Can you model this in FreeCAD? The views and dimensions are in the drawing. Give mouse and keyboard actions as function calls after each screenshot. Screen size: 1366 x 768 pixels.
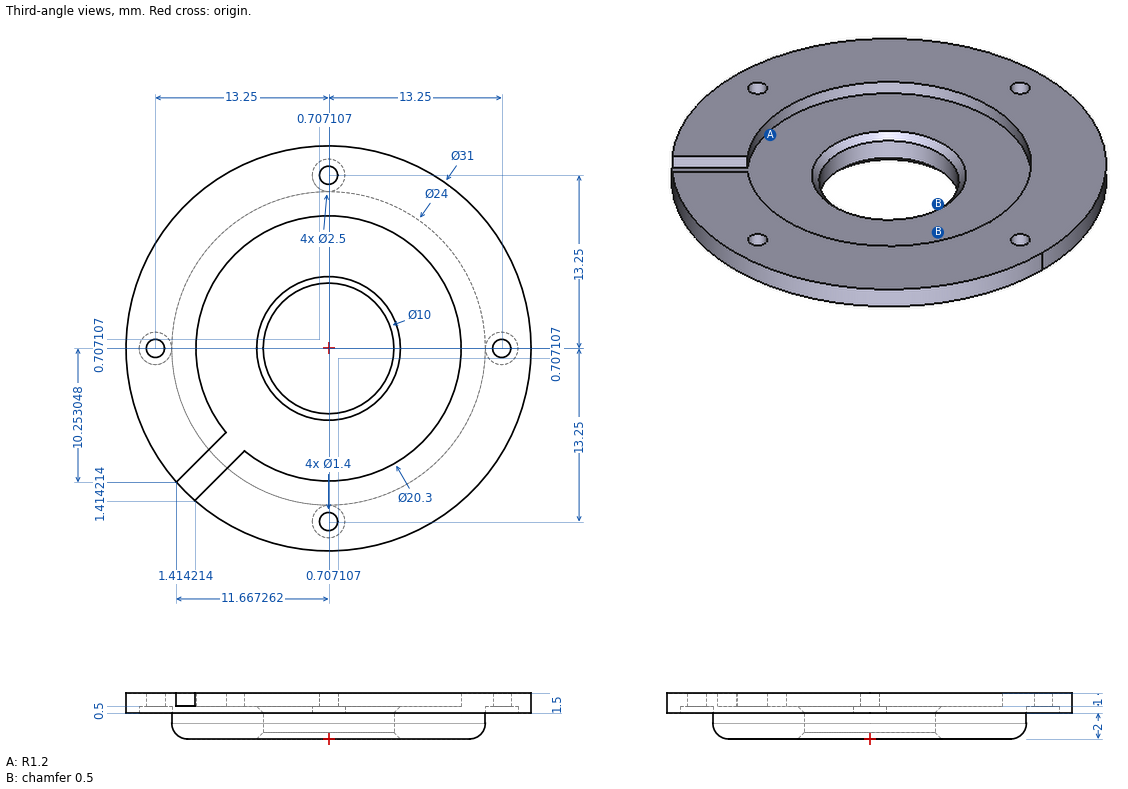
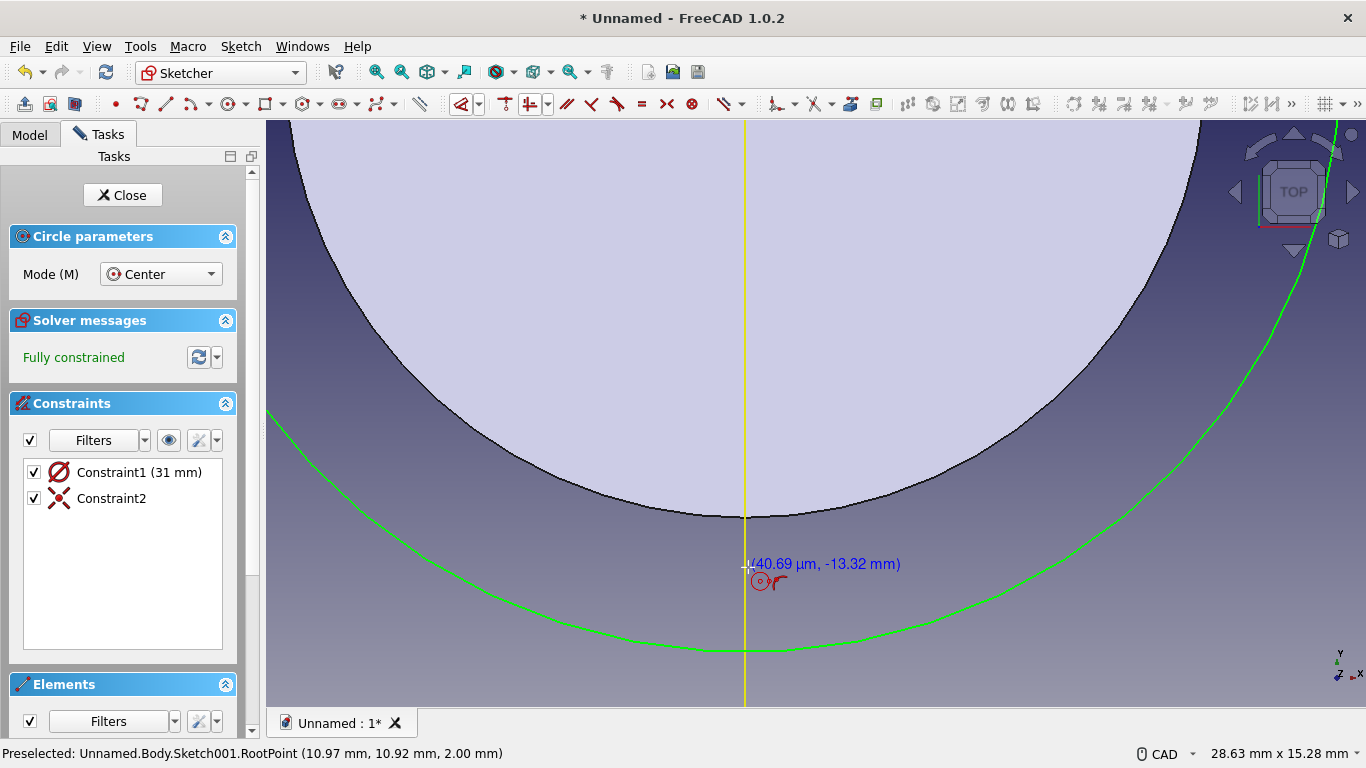
click(745, 566)
move(764, 547)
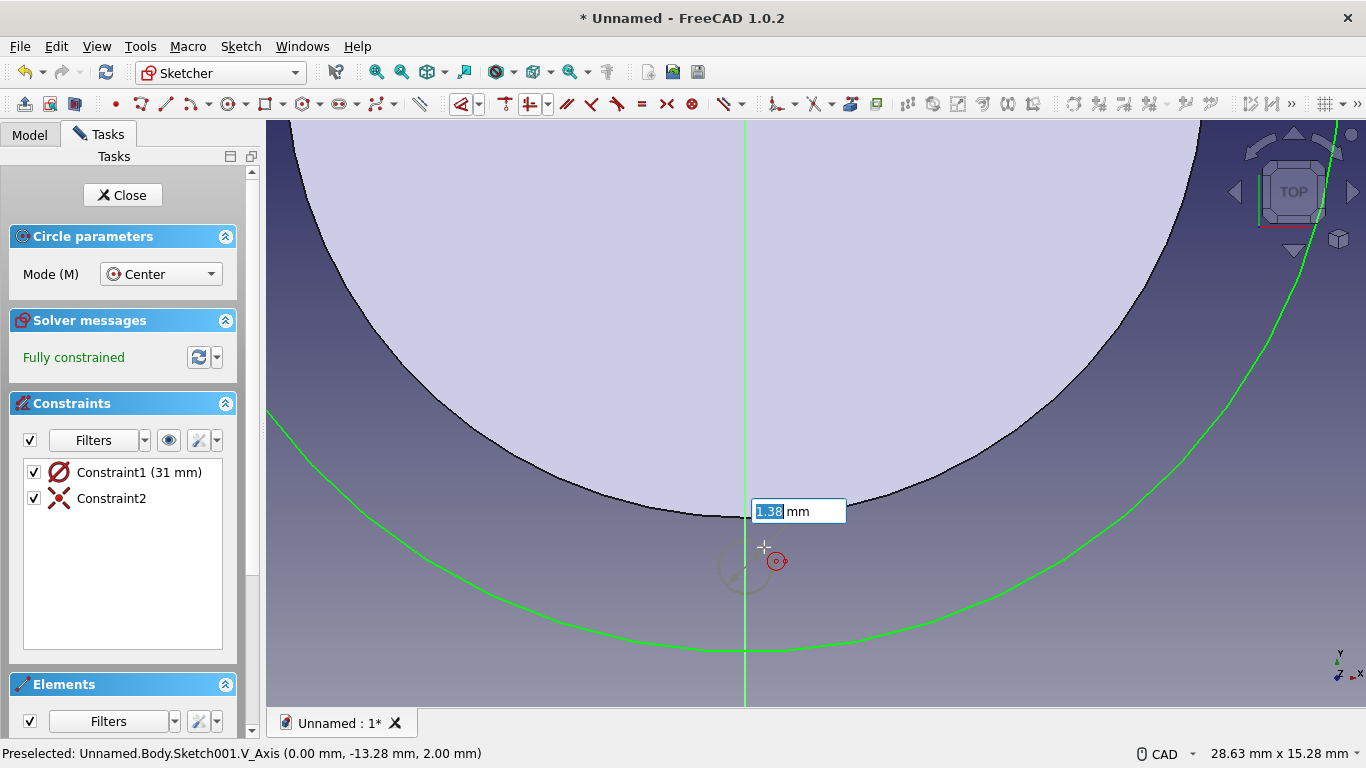
text(1.4)
key(Return)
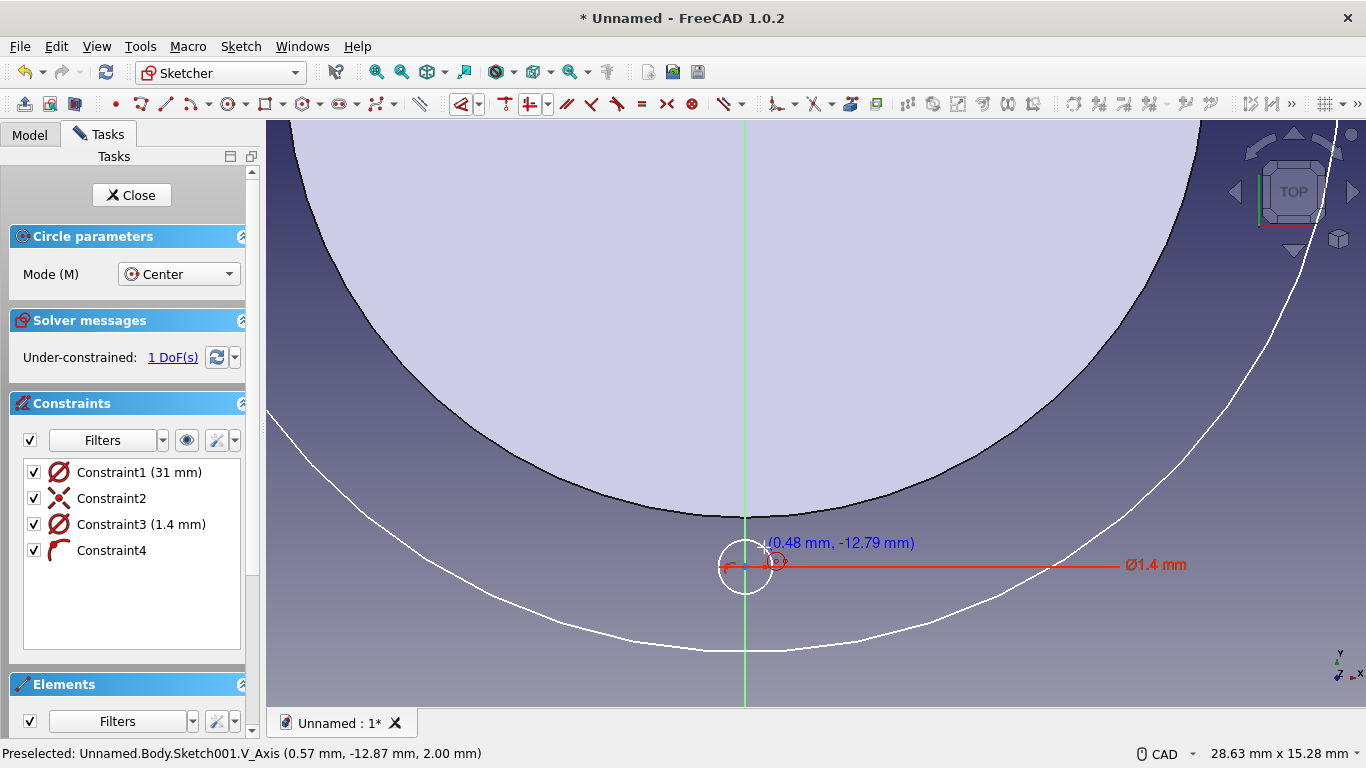
scroll(748, 567, down, 6)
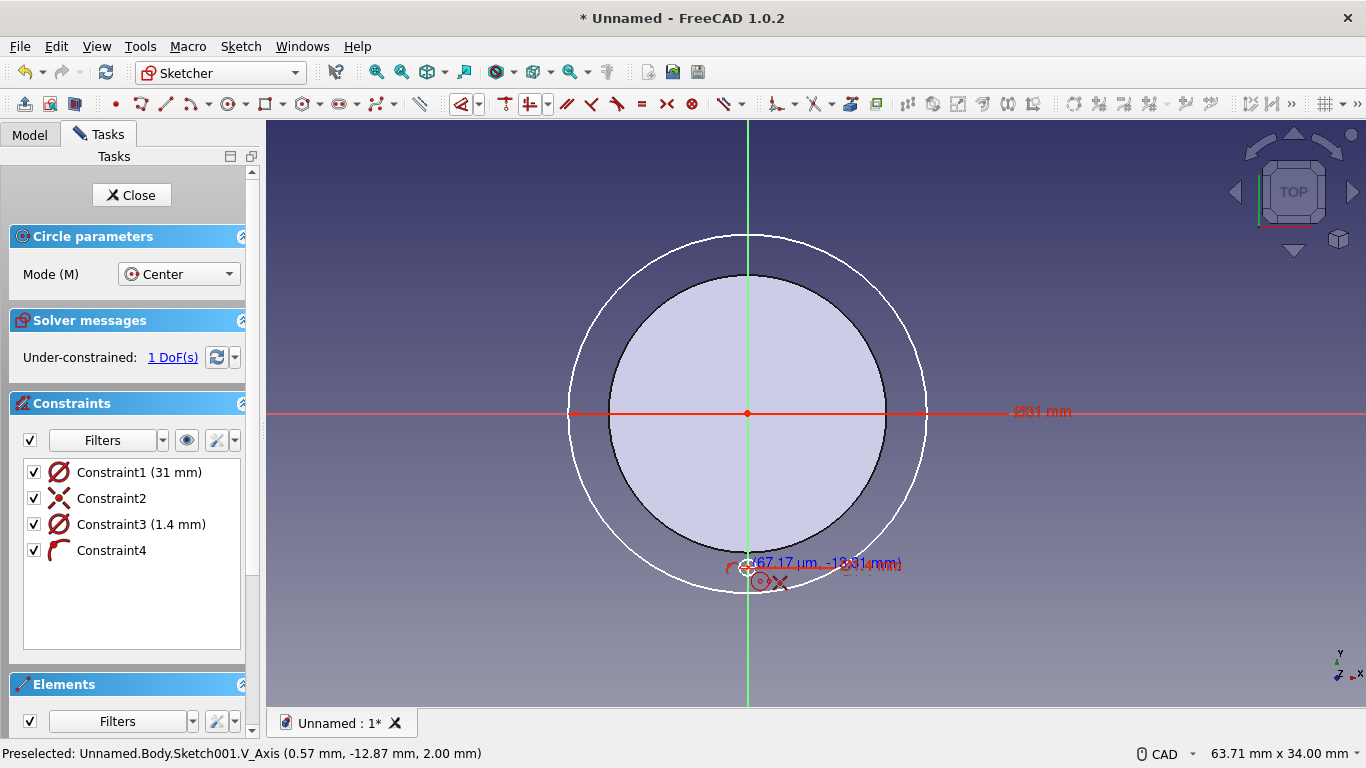
scroll(594, 414, up, 6)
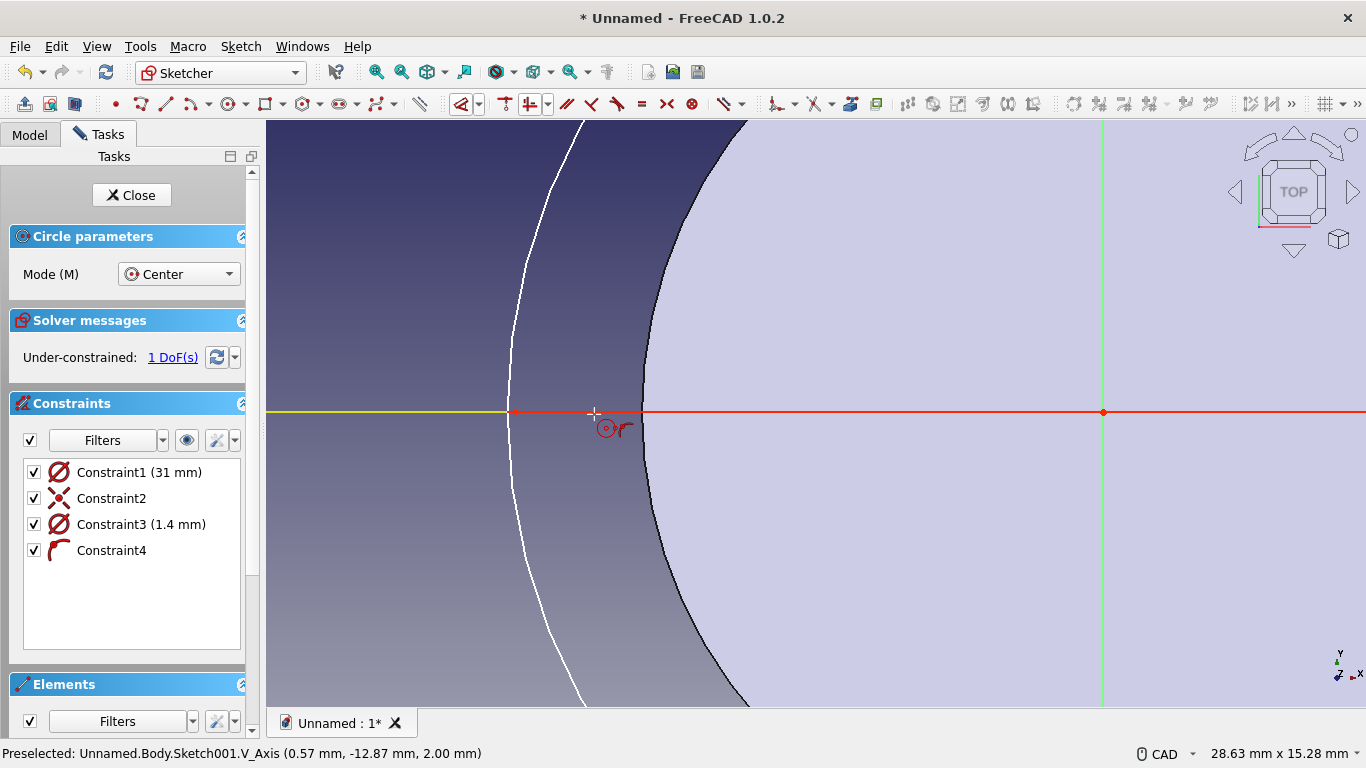
click(594, 412)
move(613, 393)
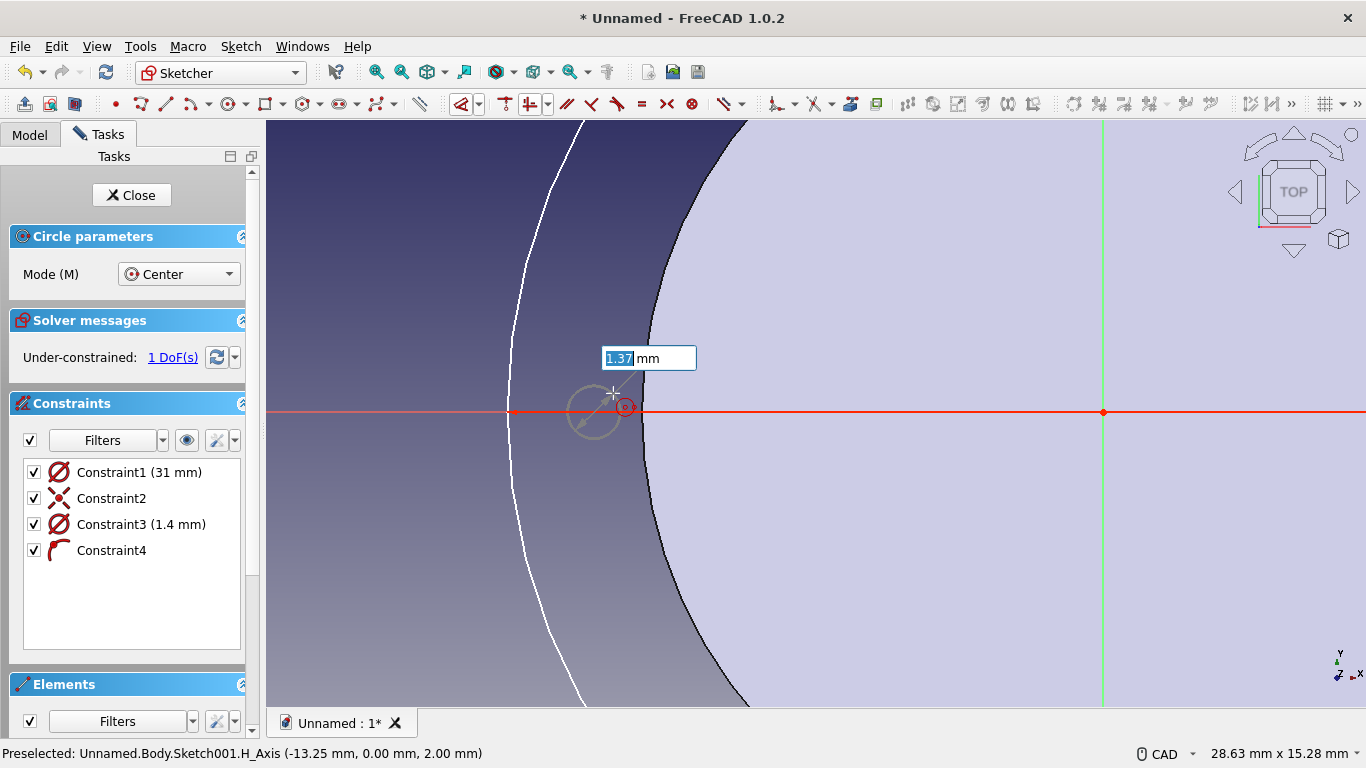
text(1.4)
key(Return)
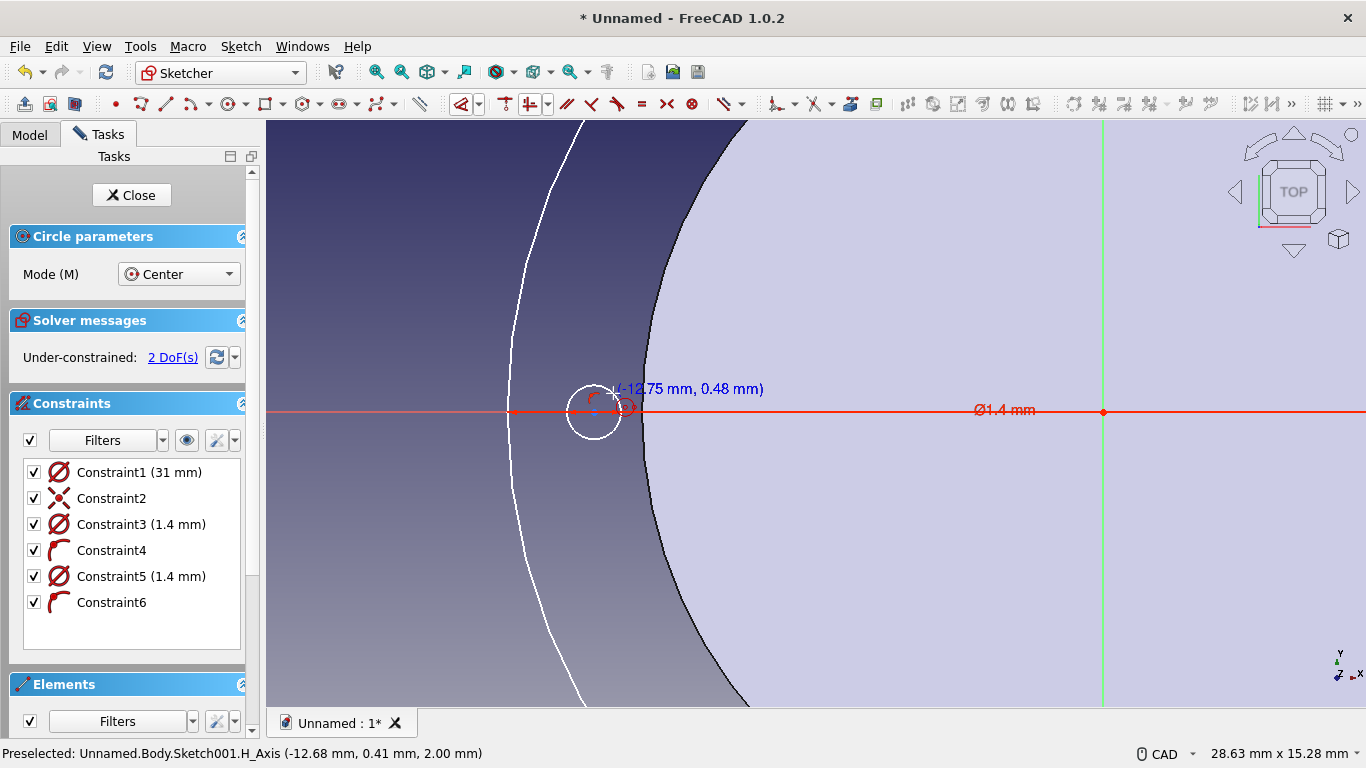
scroll(594, 414, down, 6)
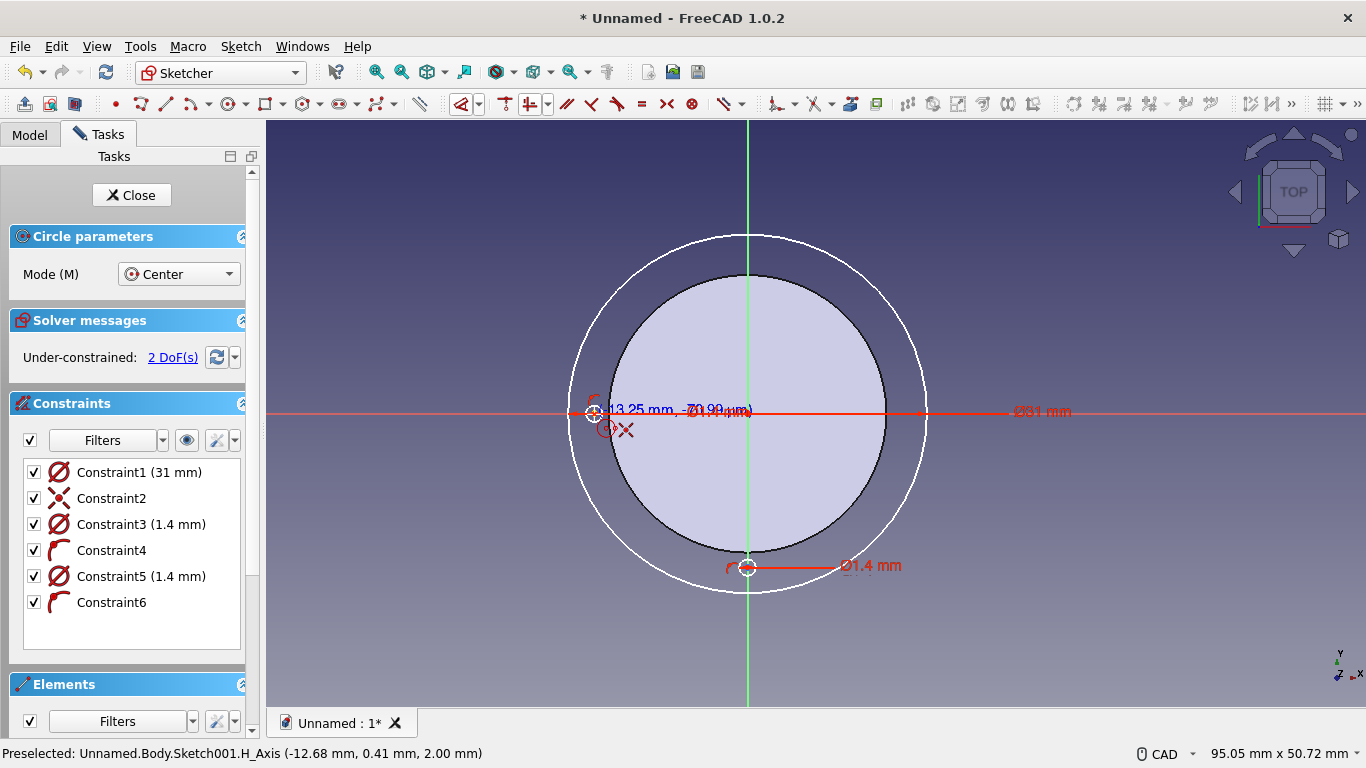
scroll(901, 414, up, 6)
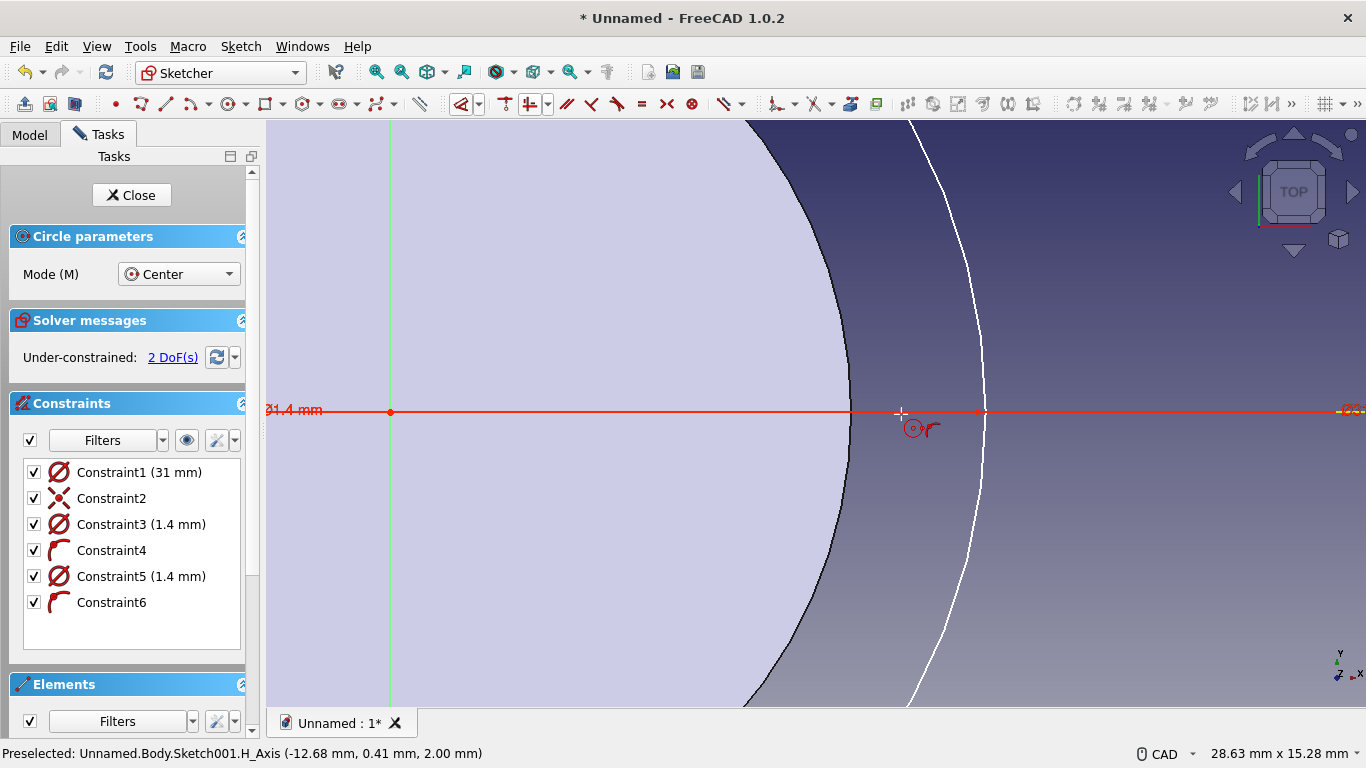
click(899, 412)
move(918, 393)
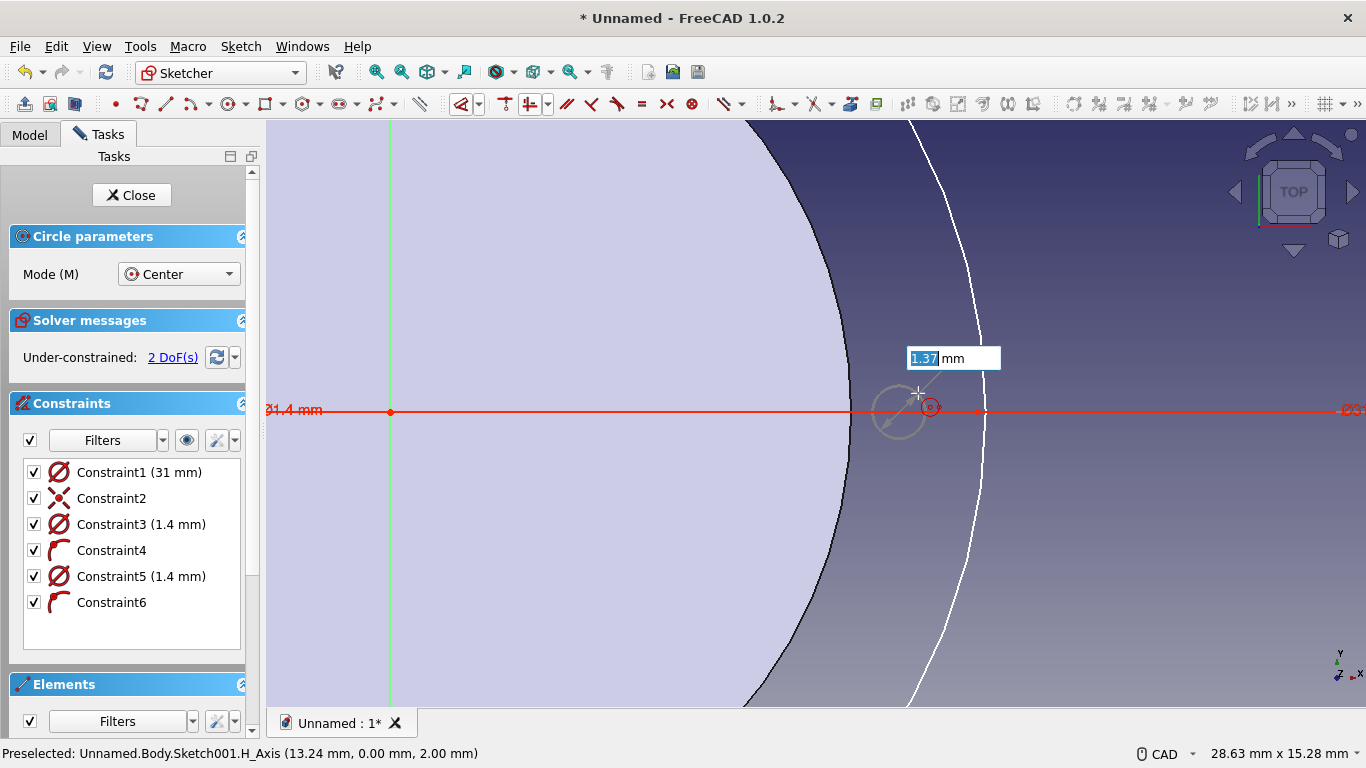
text(1.4)
key(Return)